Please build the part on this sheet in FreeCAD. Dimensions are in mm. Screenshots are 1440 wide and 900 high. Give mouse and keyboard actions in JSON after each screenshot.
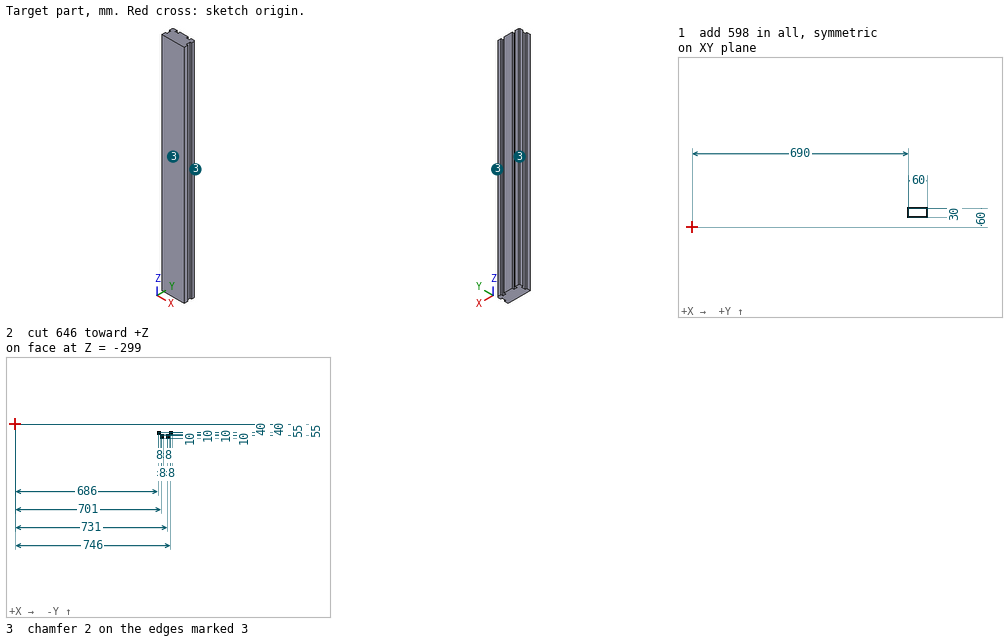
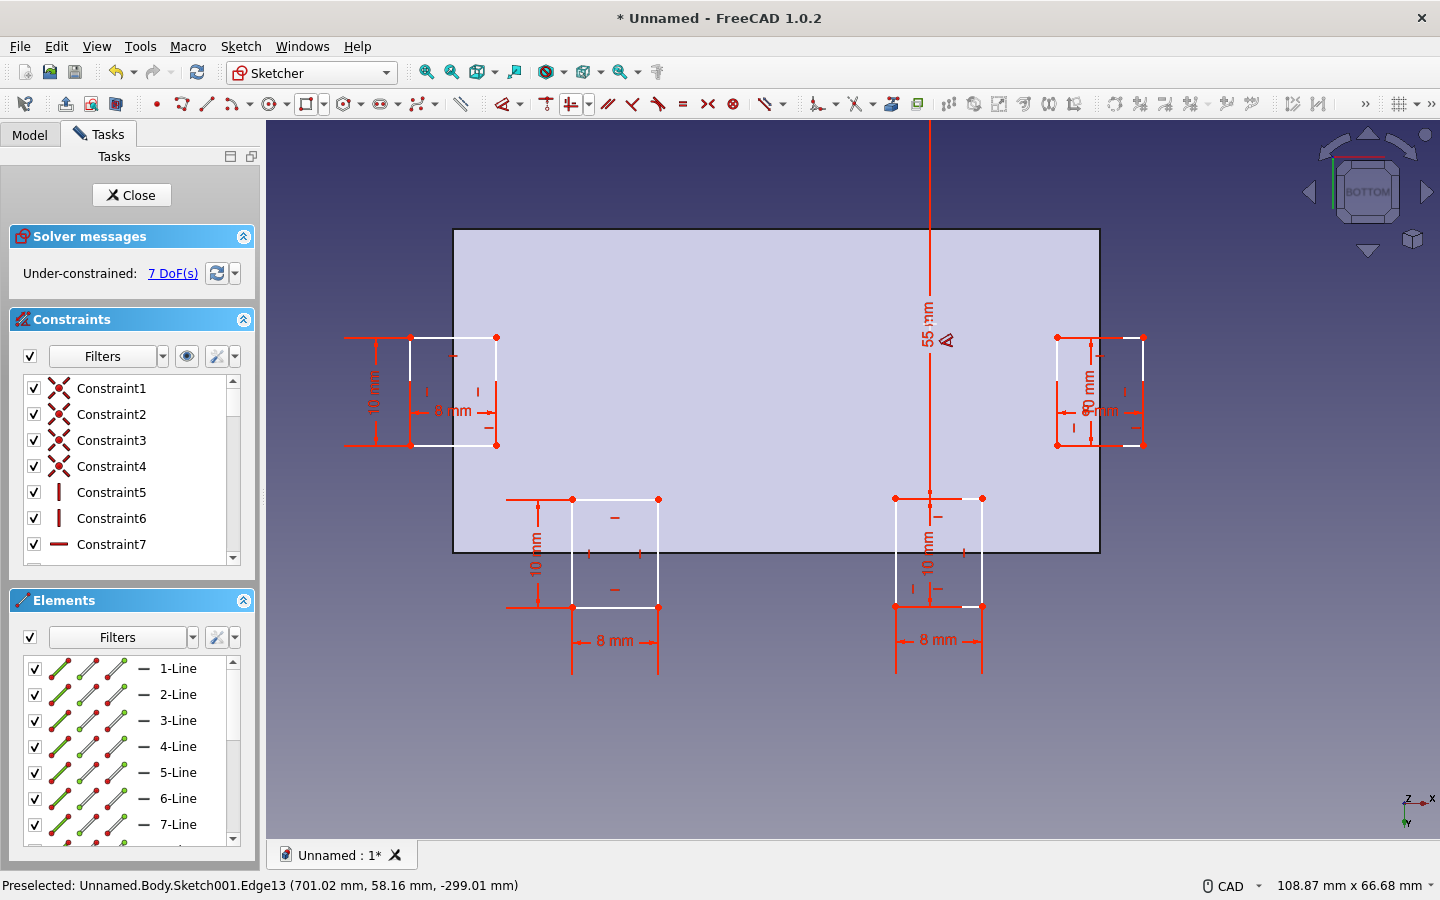
{"action": "left_click", "coordinate": [1057, 338]}
{"action": "left_click", "coordinate": [1091, 243]}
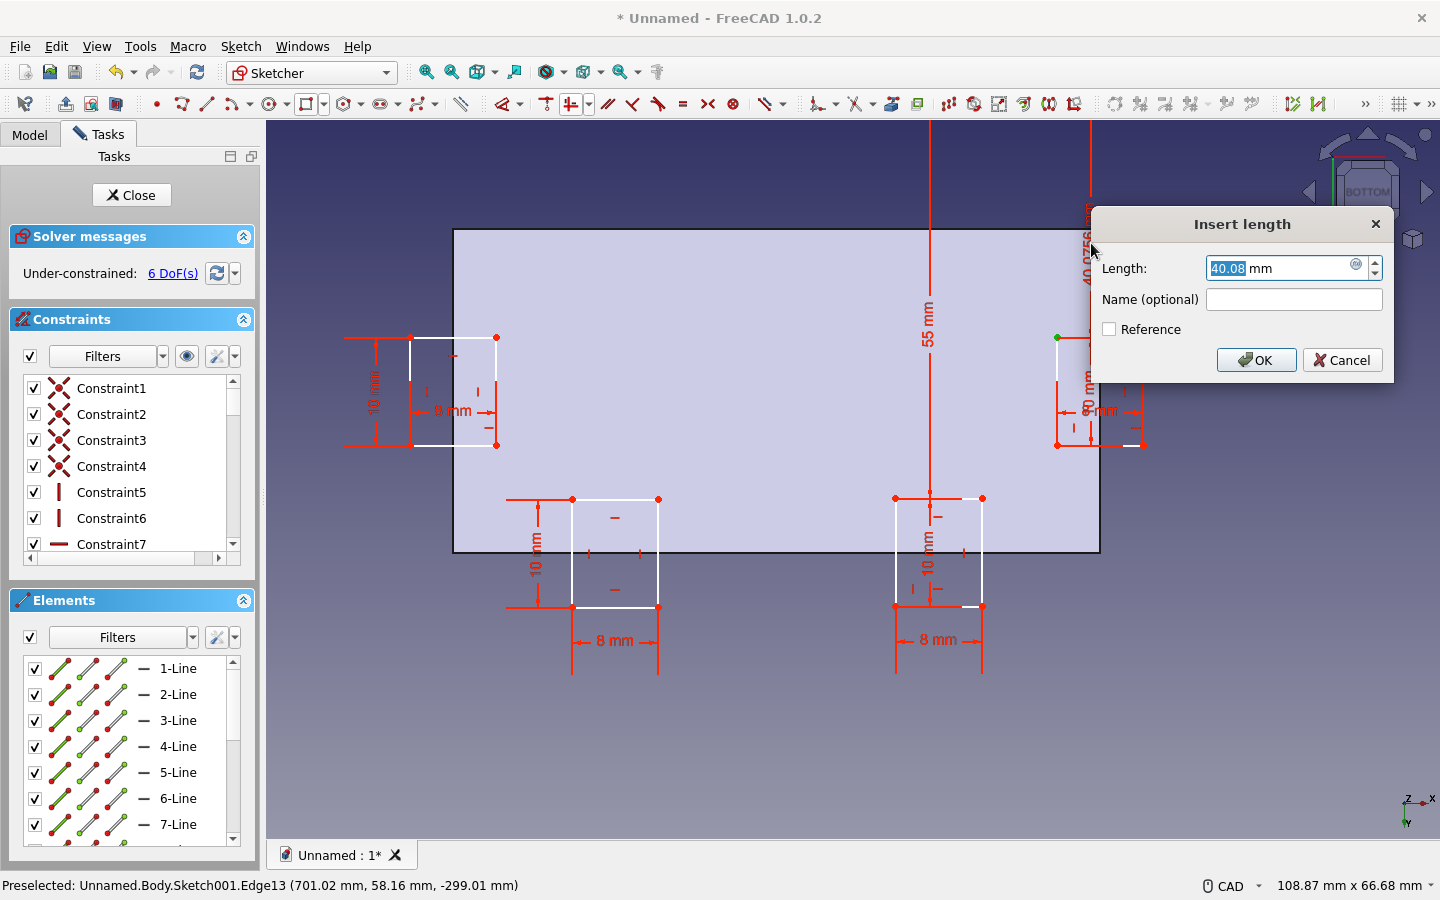
{"action": "type", "text": "40"}
{"action": "key", "text": "Return"}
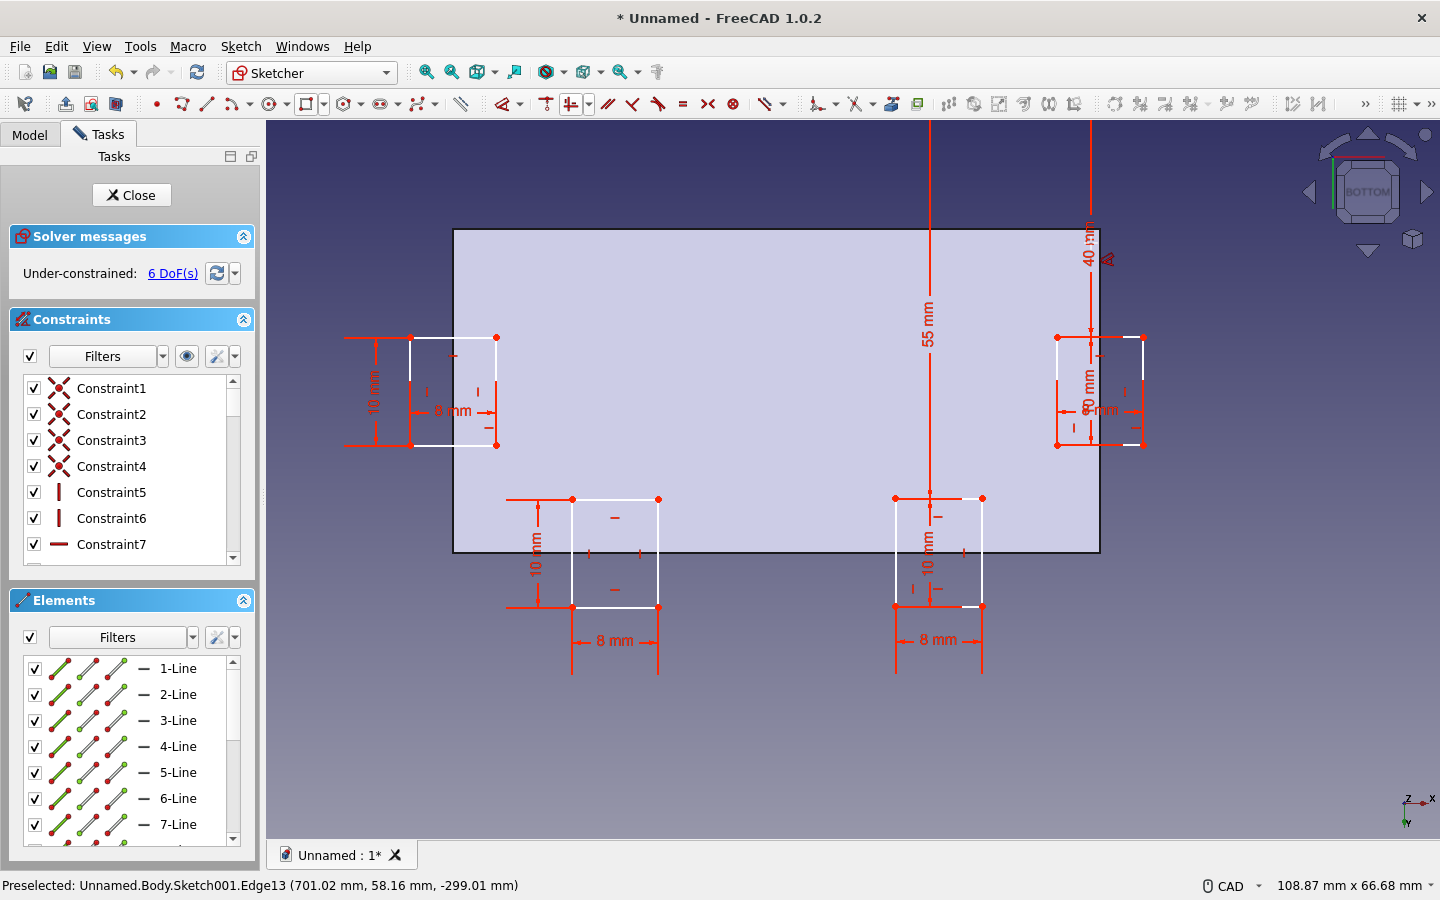
{"action": "left_click", "coordinate": [410, 338]}
{"action": "left_click", "coordinate": [444, 243]}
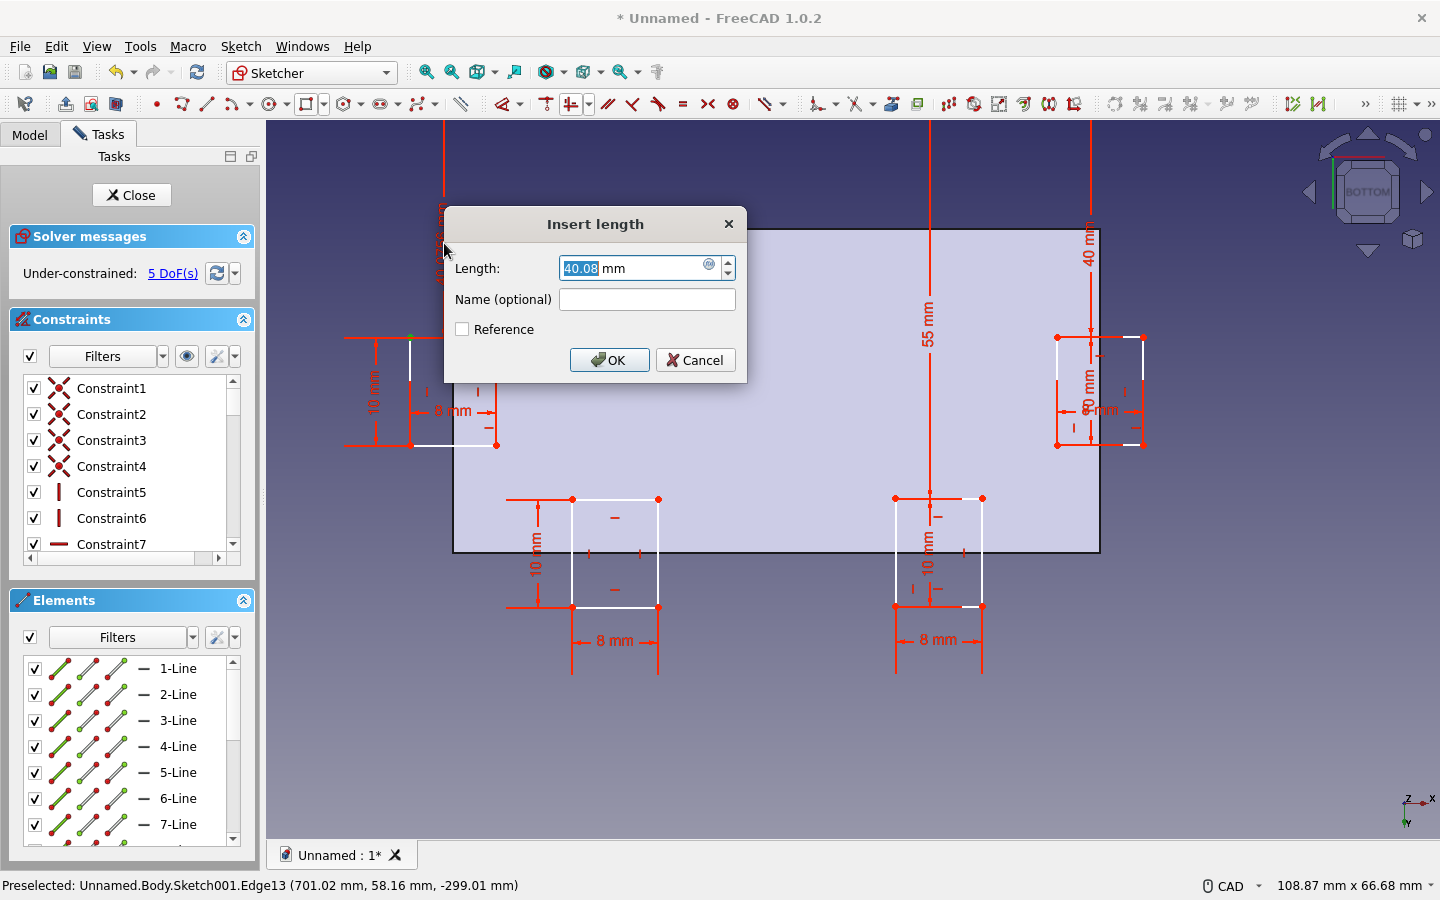
{"action": "type", "text": "40"}
{"action": "key", "text": "Return"}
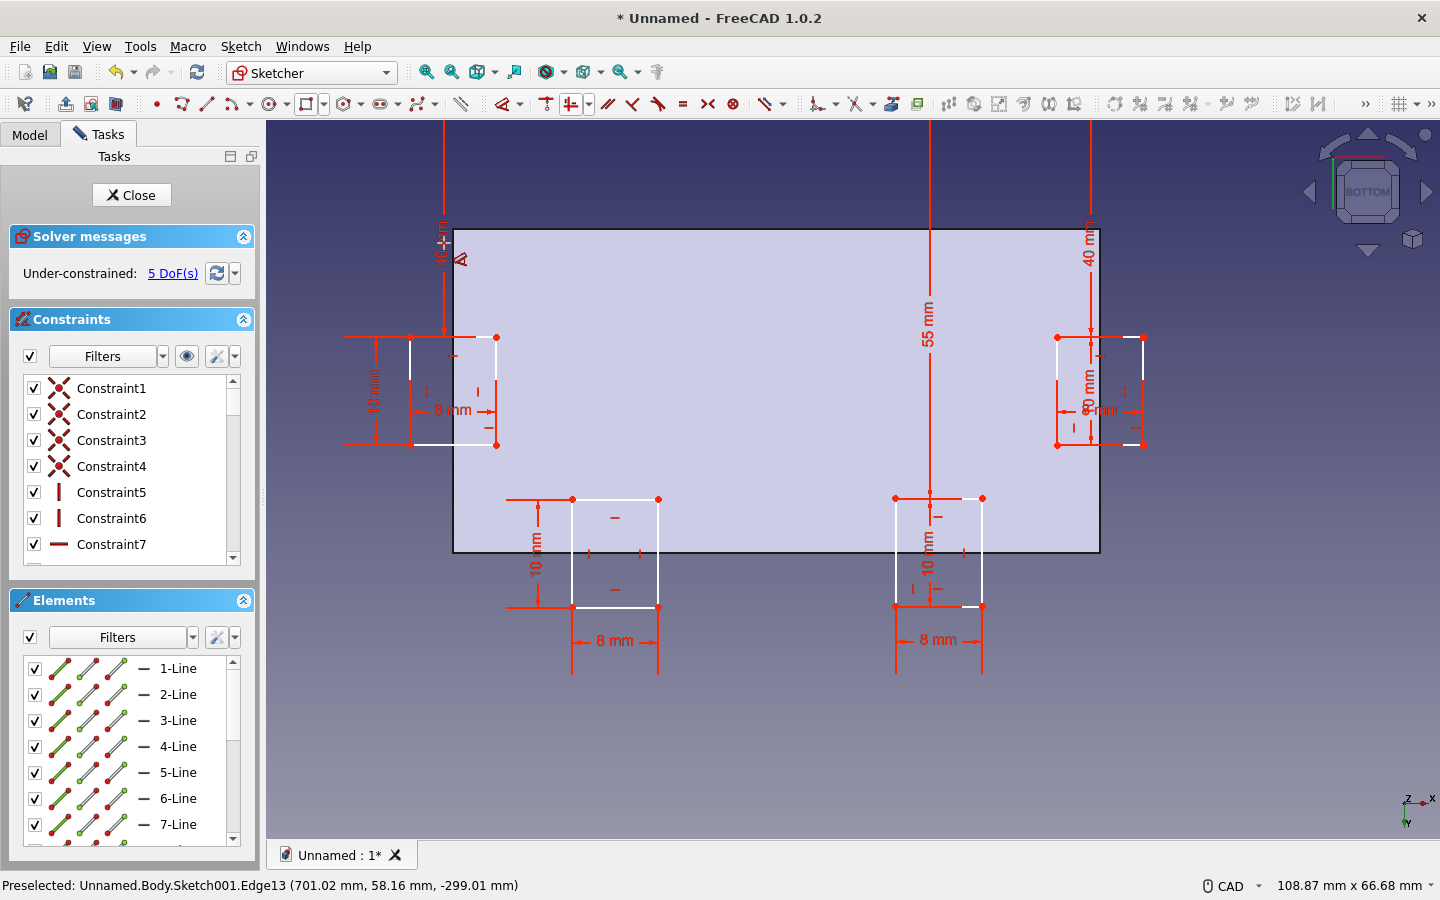
{"action": "left_click", "coordinate": [572, 500]}
{"action": "left_click", "coordinate": [606, 324]}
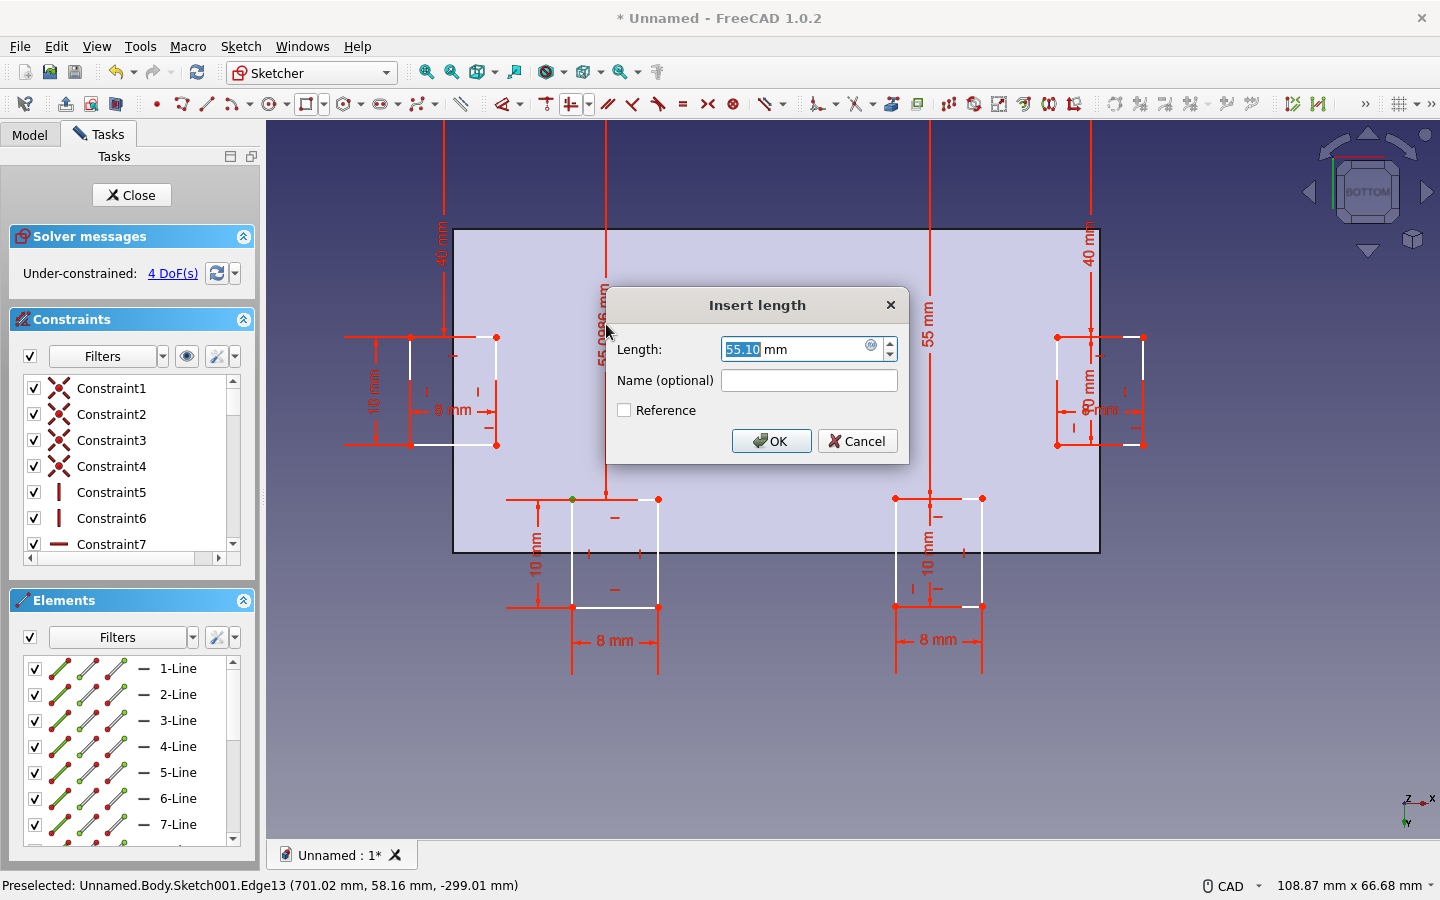
{"action": "type", "text": "55"}
{"action": "key", "text": "Return"}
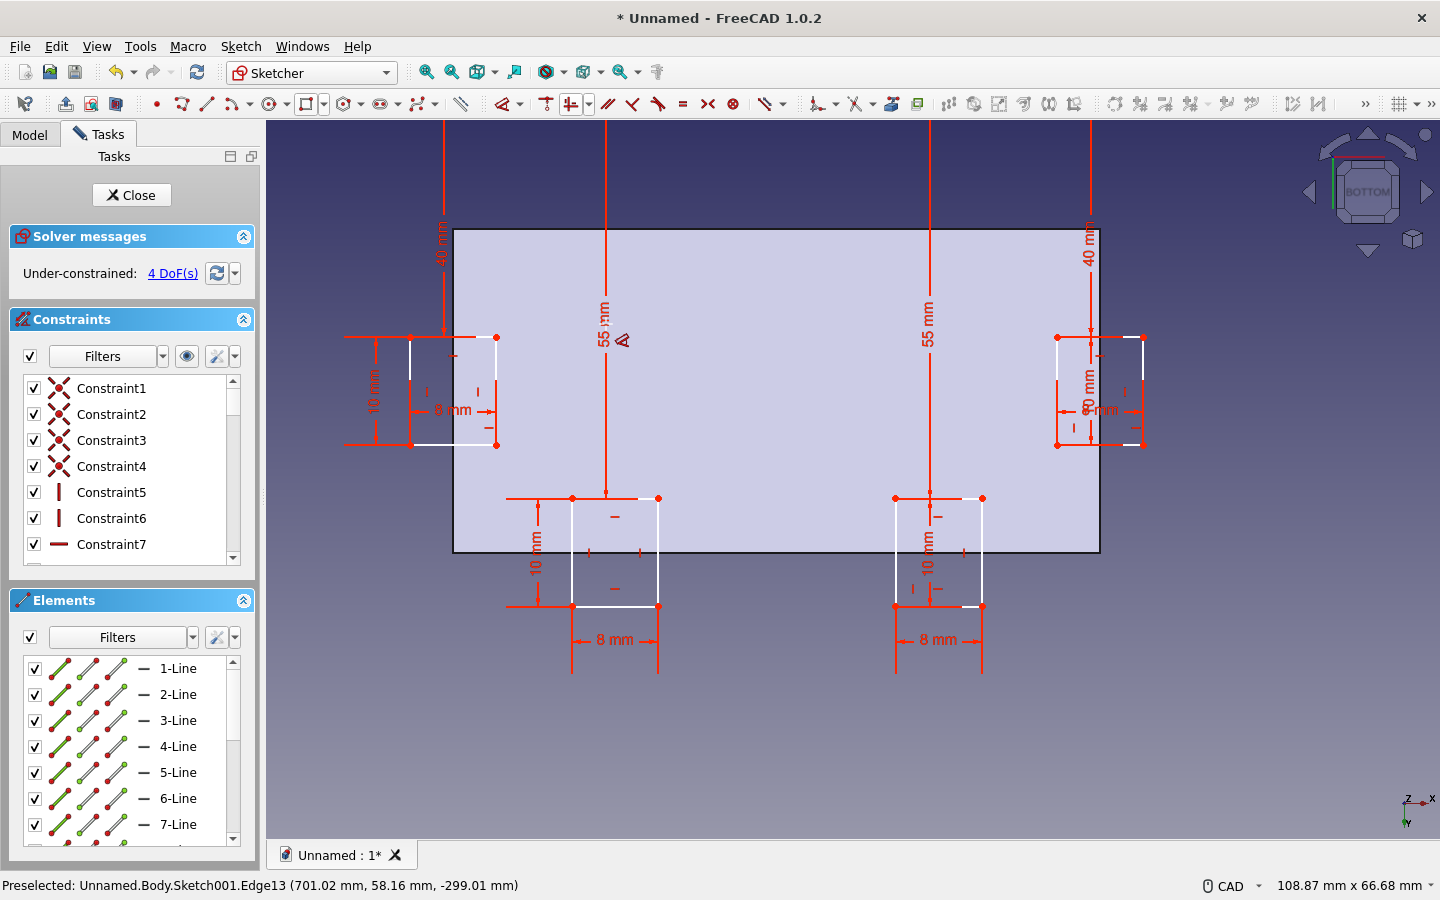
{"action": "left_click", "coordinate": [896, 499]}
{"action": "left_click", "coordinate": [595, 533]}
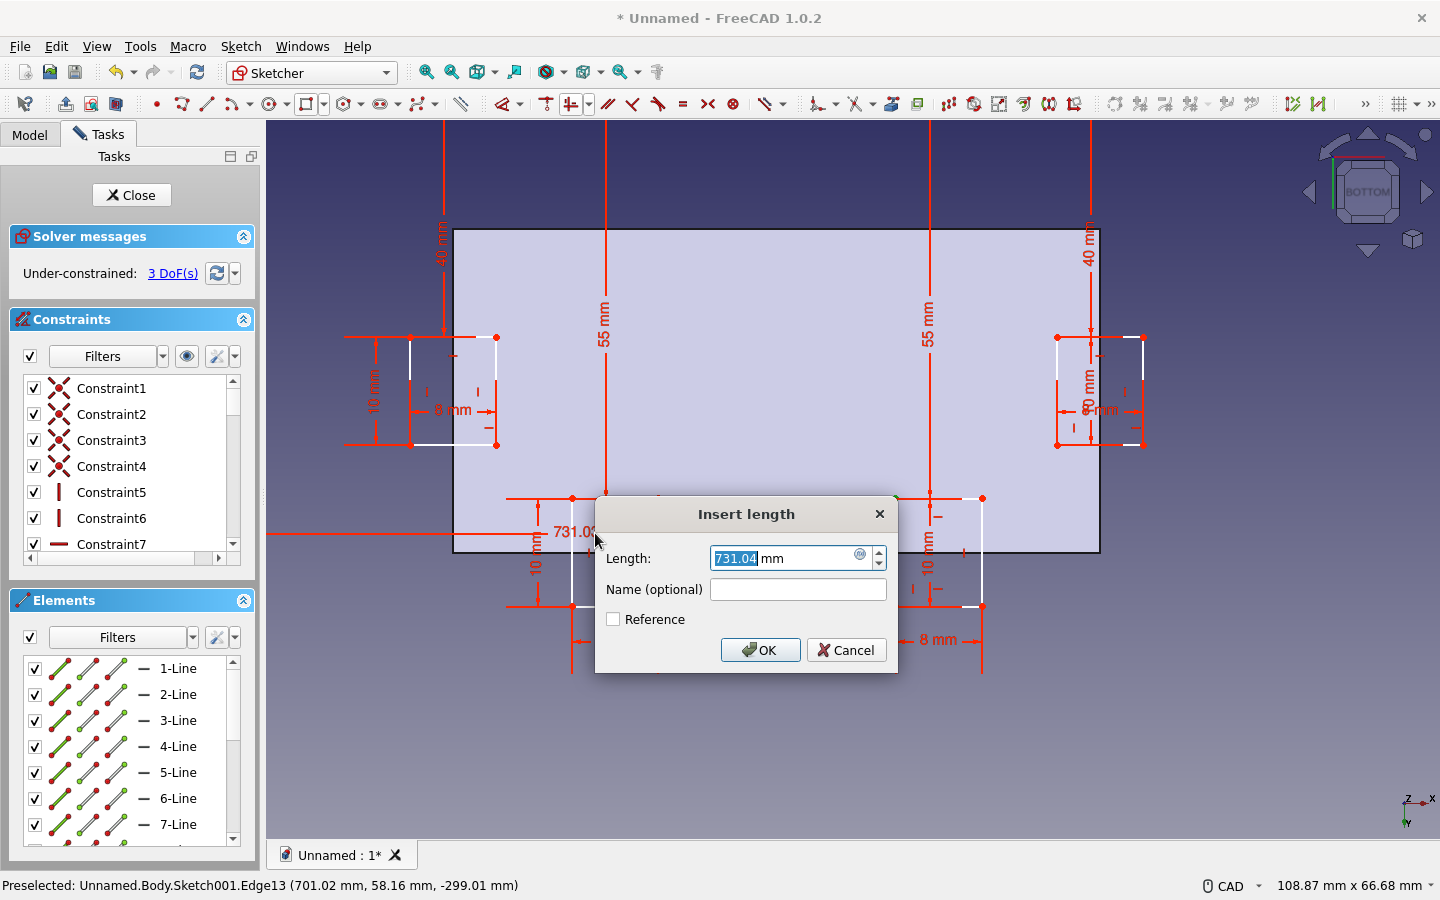
{"action": "type", "text": "731"}
{"action": "key", "text": "Return"}